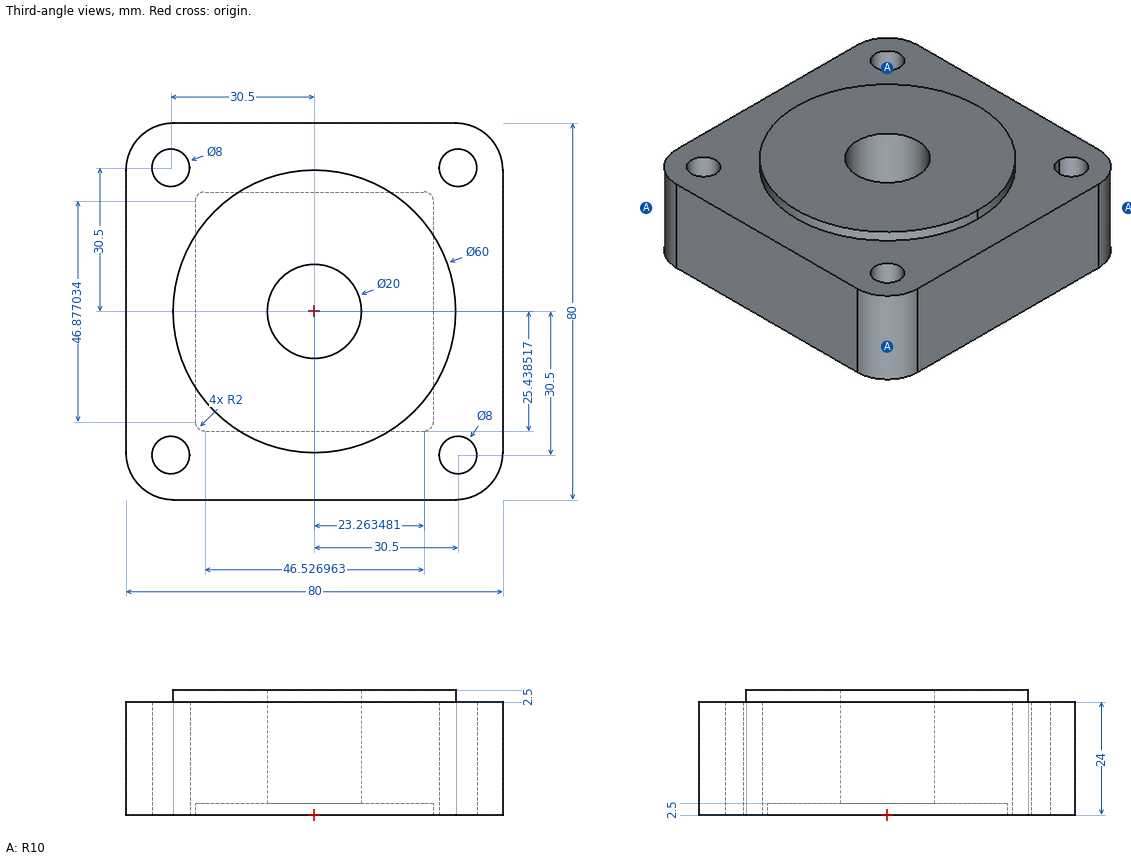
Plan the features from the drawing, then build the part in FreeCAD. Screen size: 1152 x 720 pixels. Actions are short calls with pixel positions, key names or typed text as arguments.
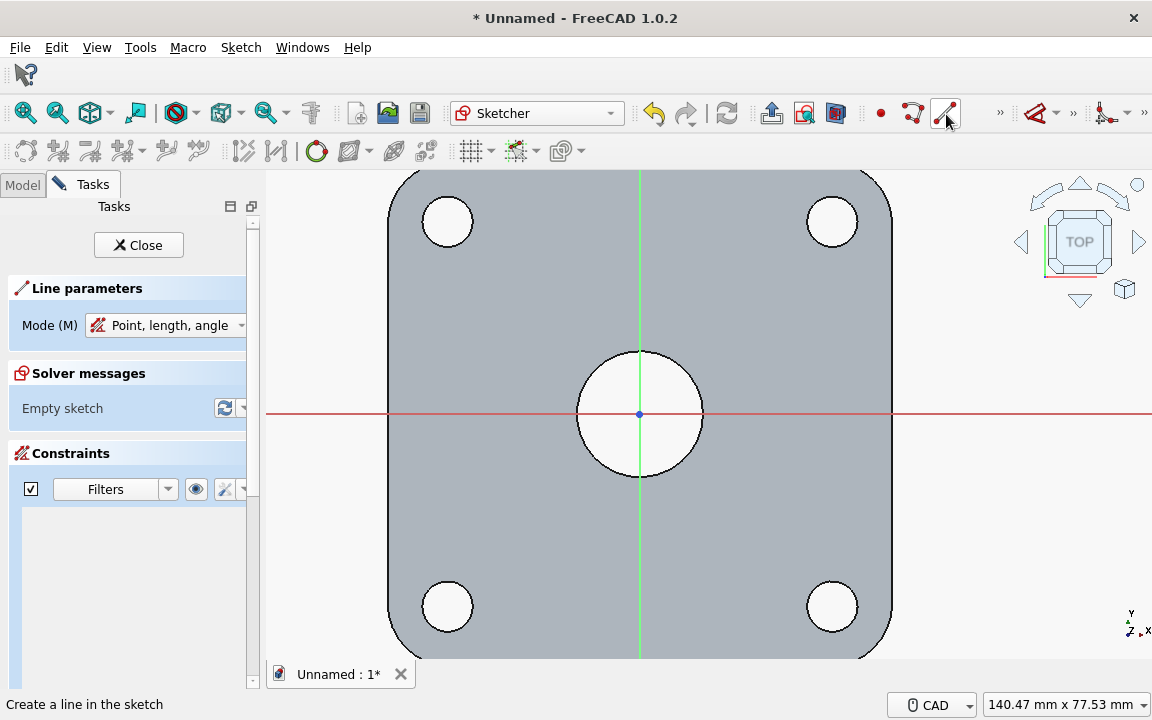
click(787, 575)
click(493, 575)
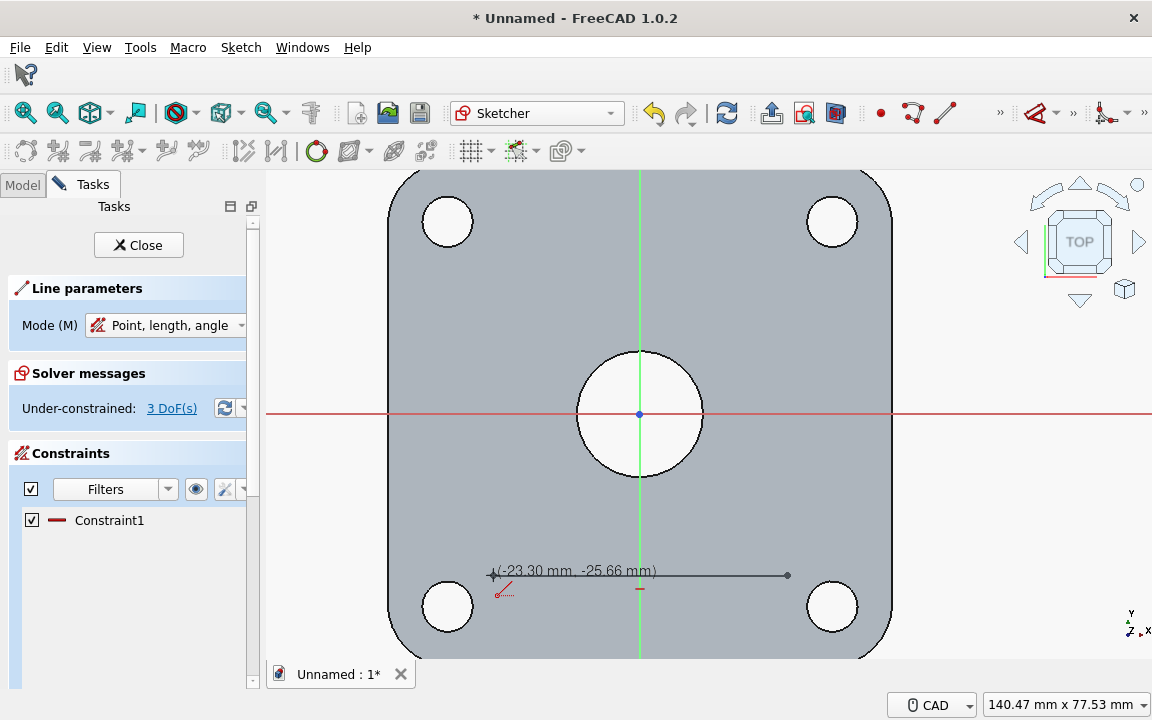
click(481, 562)
click(481, 266)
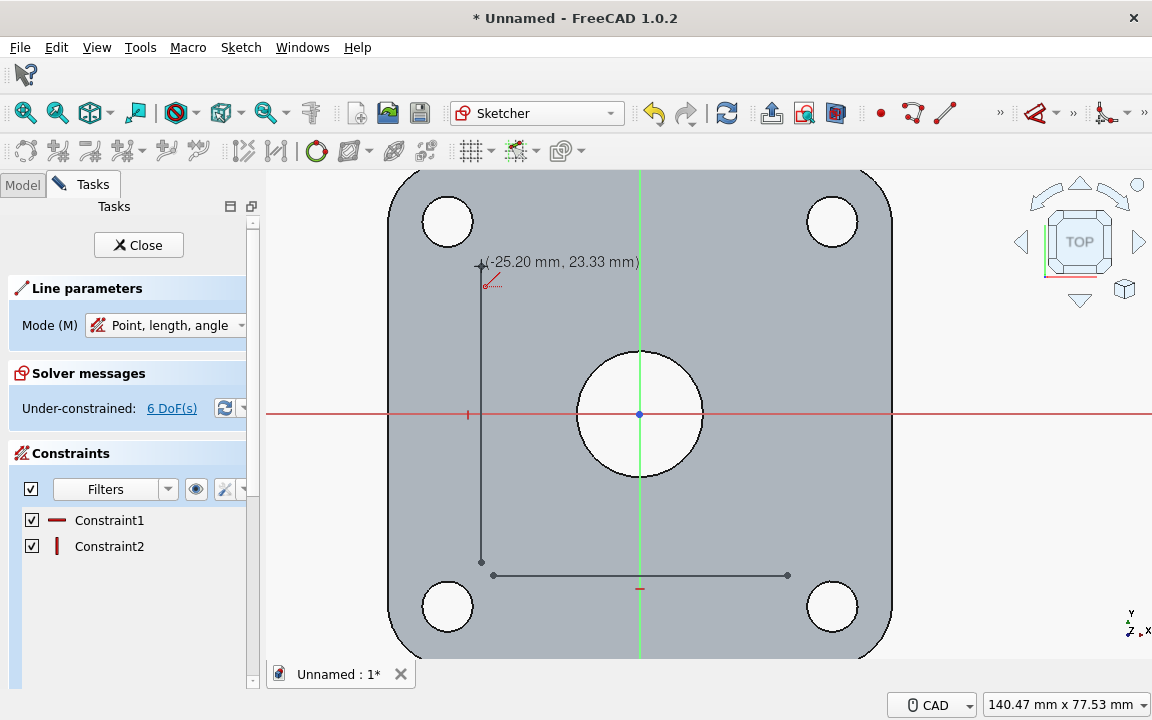
click(493, 254)
click(787, 254)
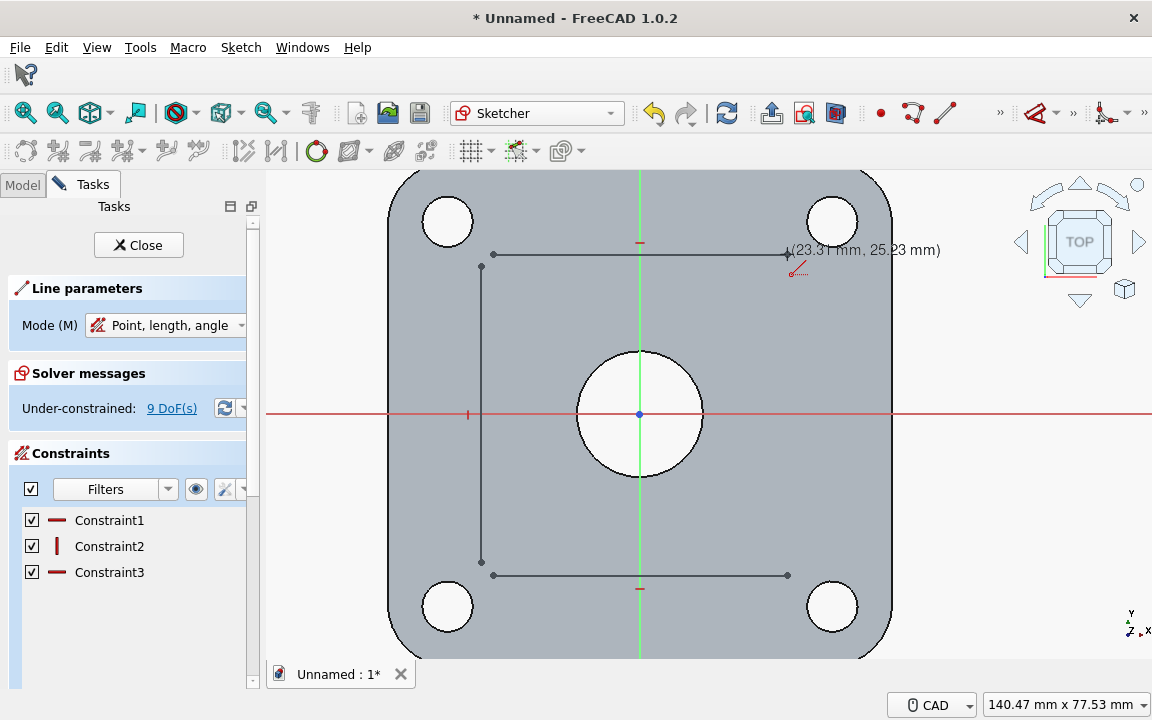
click(799, 266)
click(799, 562)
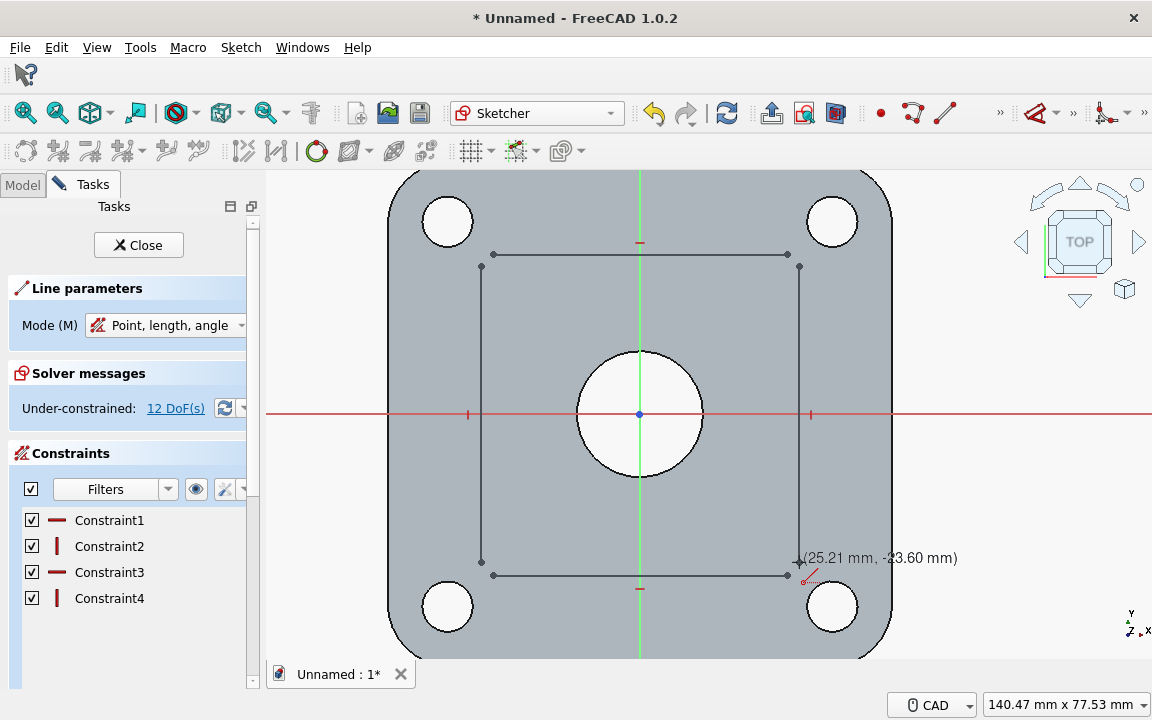
key(g)
key(3)
key(a)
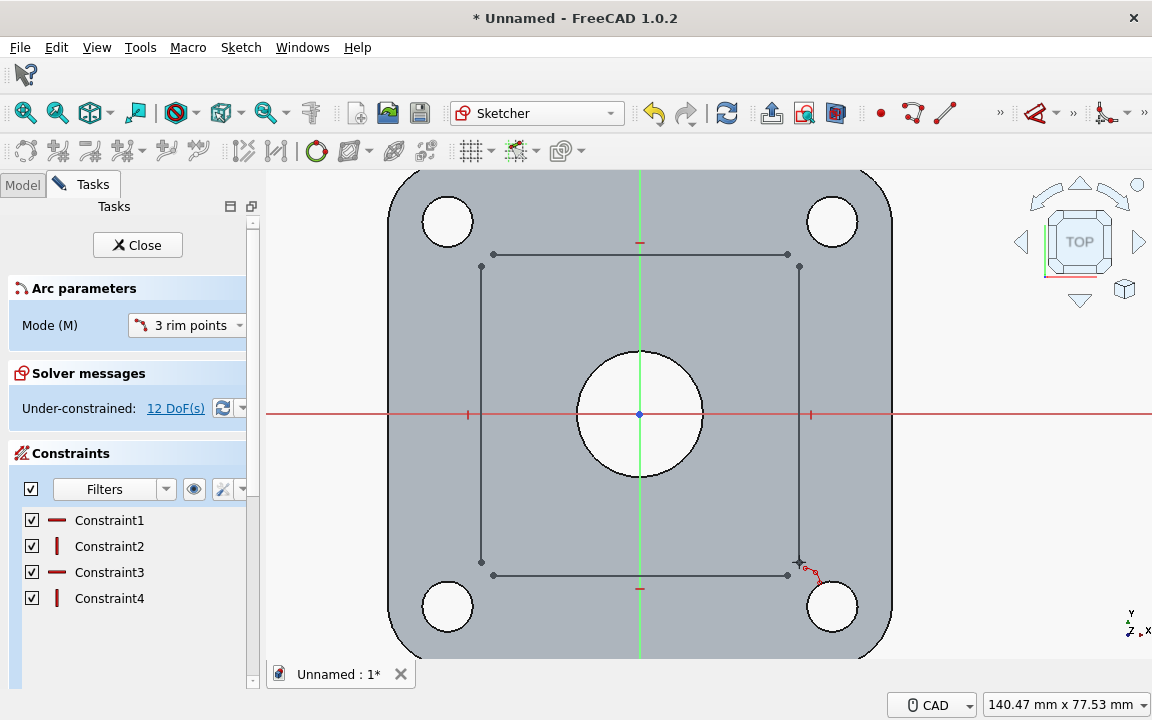
click(493, 576)
click(481, 563)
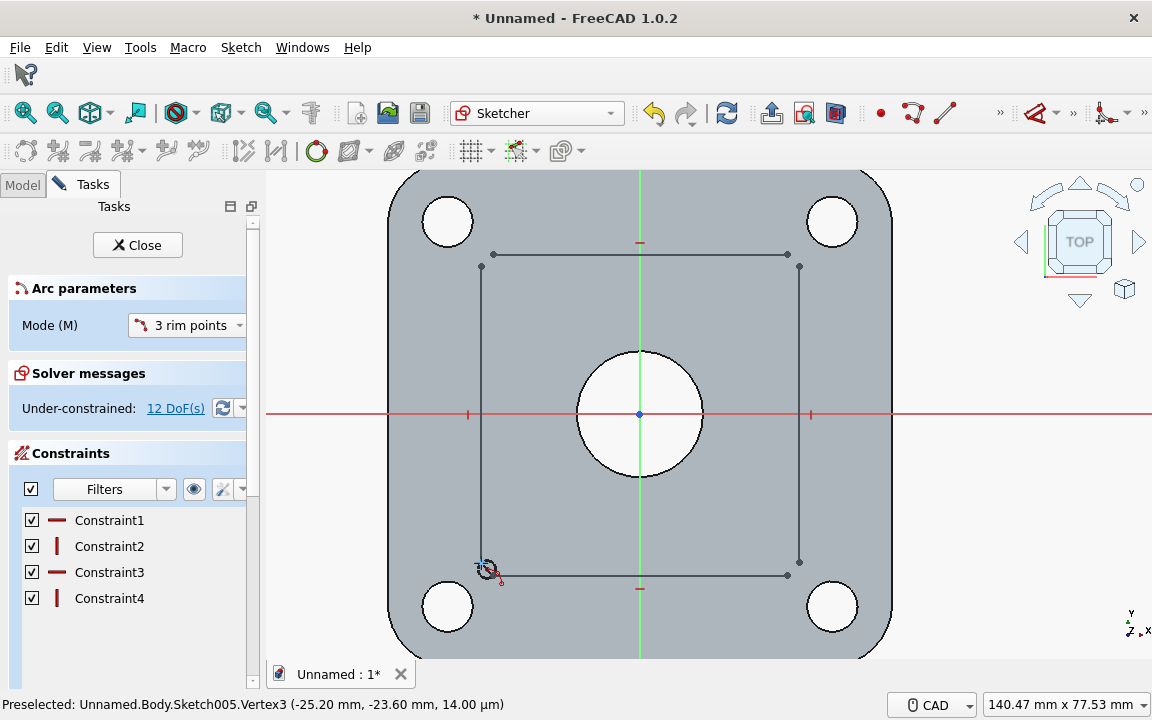
scroll(484, 571, up, 8)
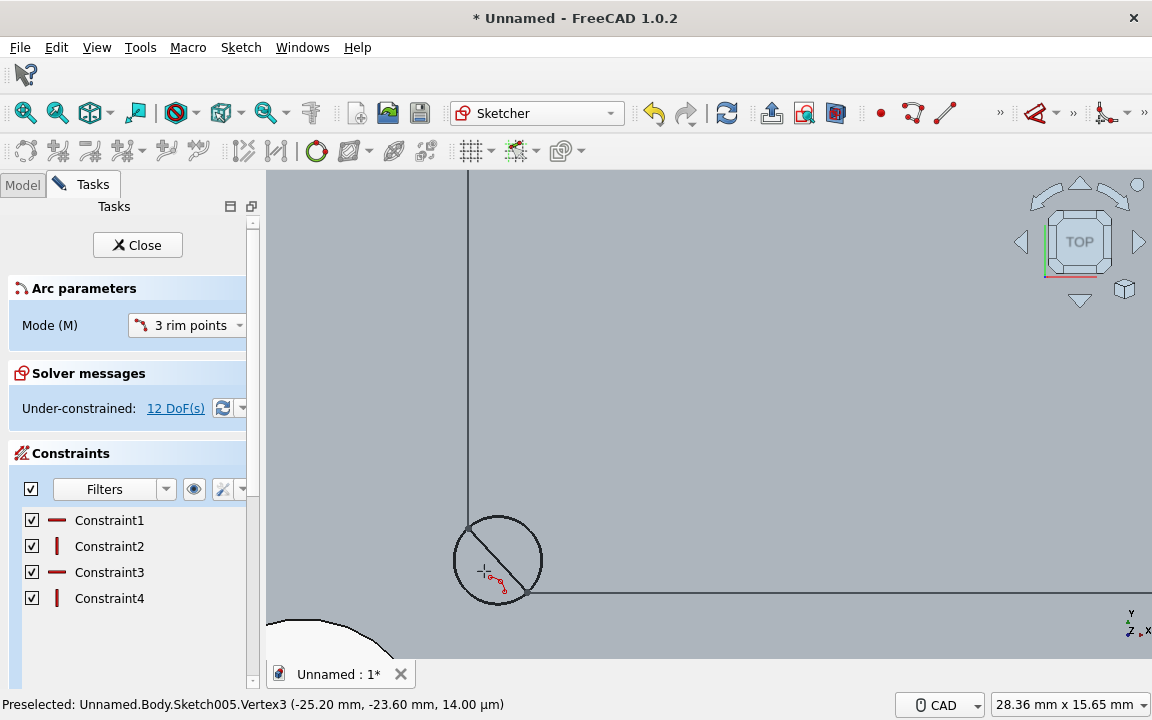
click(485, 567)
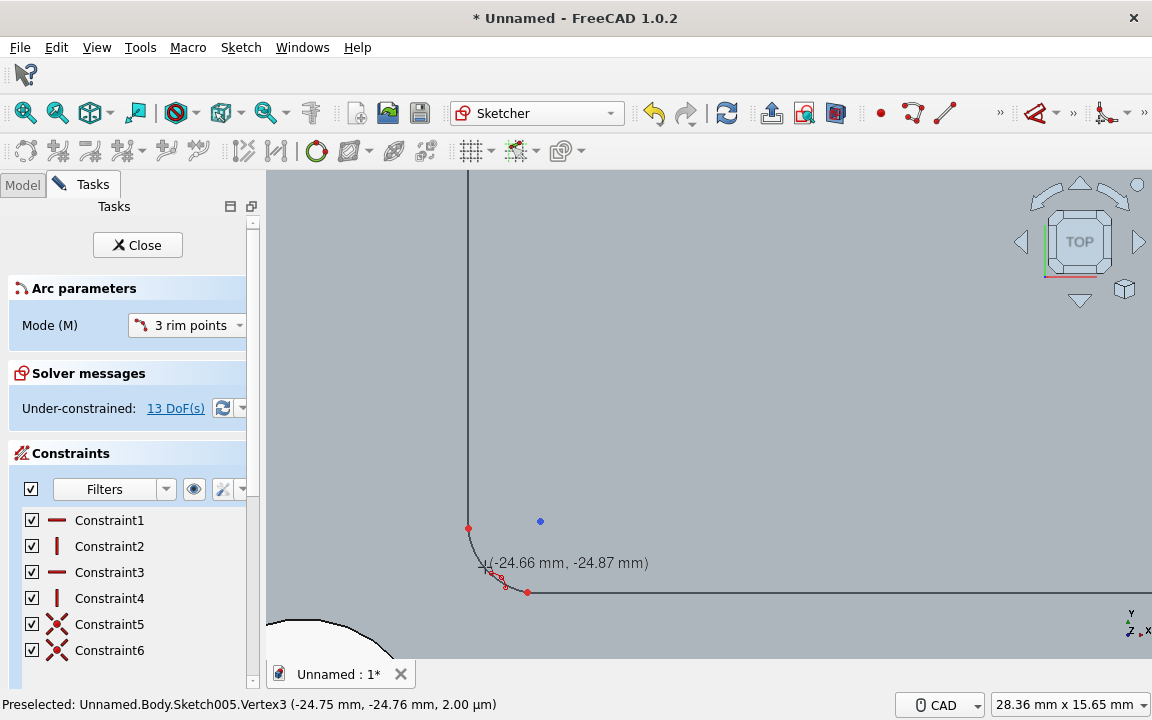
scroll(485, 572, down, 8)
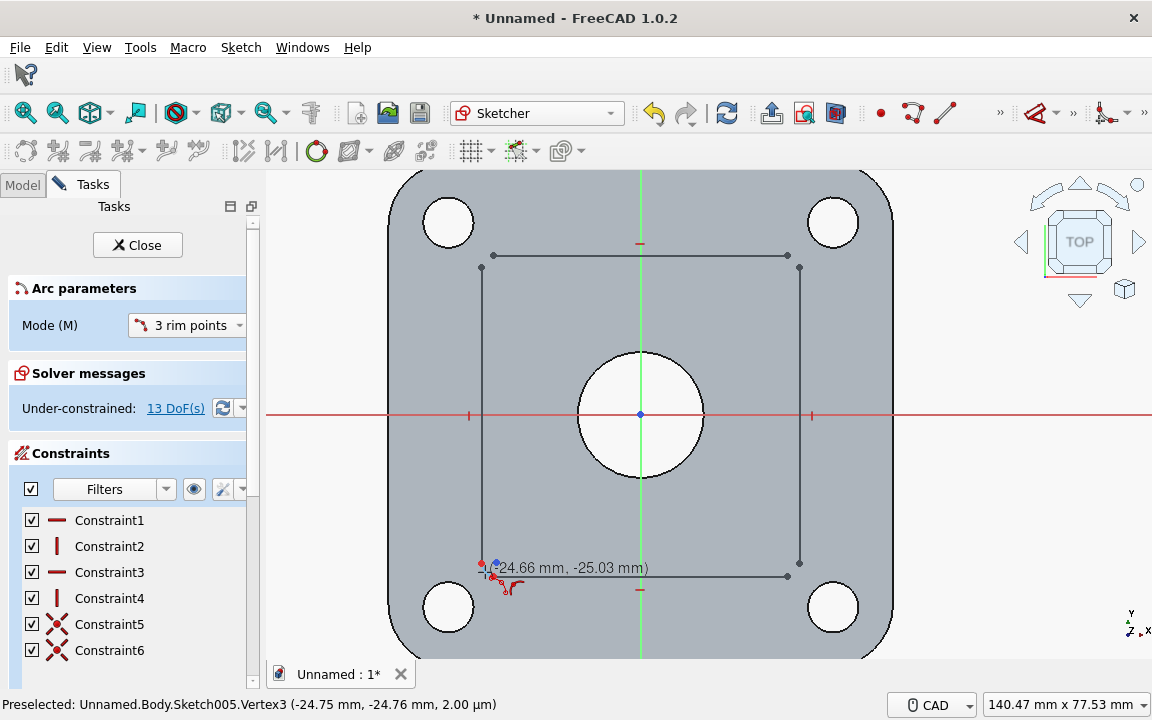
click(482, 268)
click(494, 256)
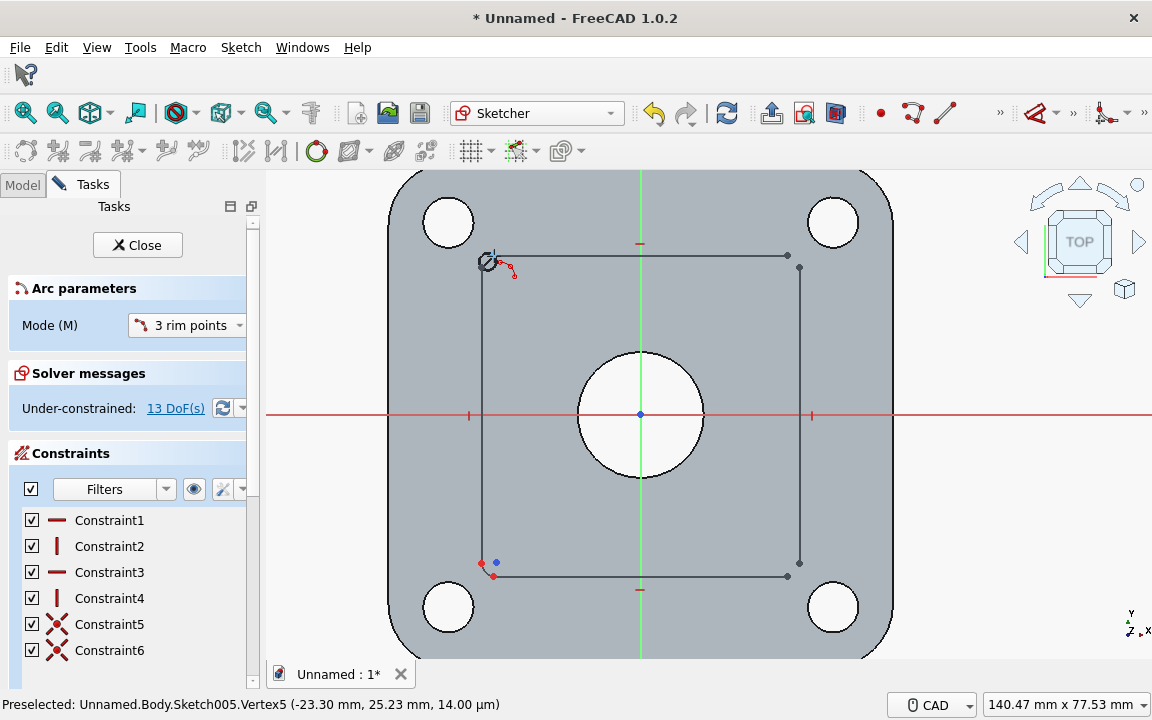
scroll(485, 258, up, 8)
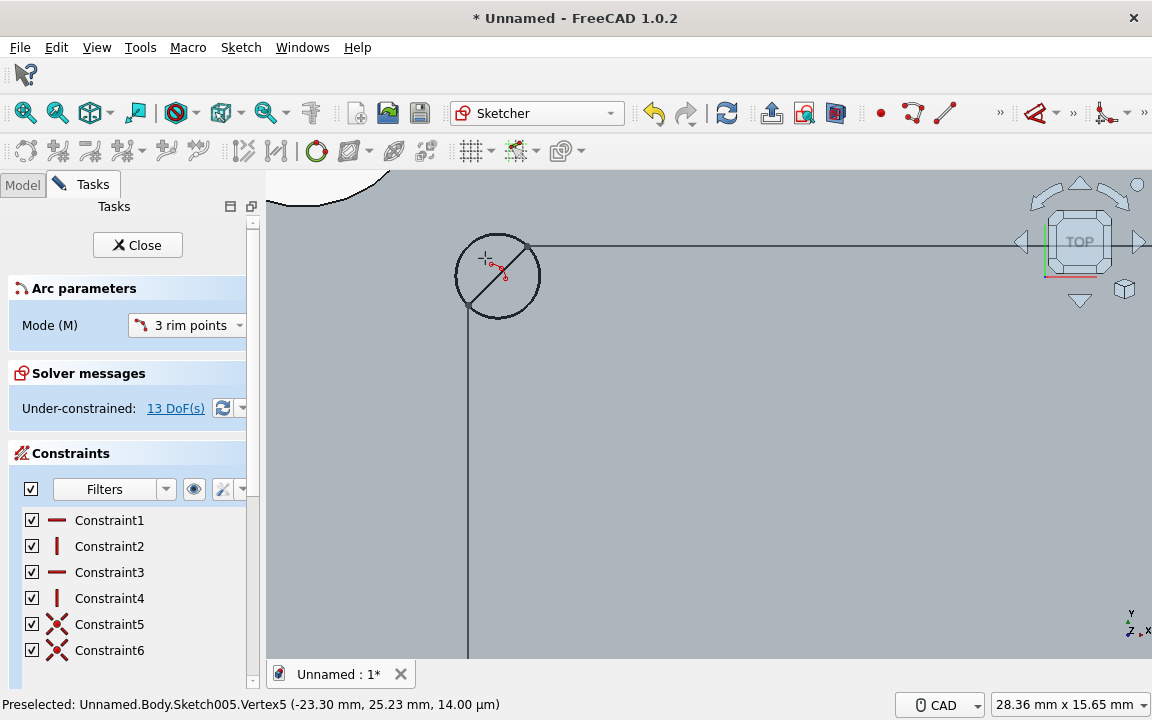
click(485, 258)